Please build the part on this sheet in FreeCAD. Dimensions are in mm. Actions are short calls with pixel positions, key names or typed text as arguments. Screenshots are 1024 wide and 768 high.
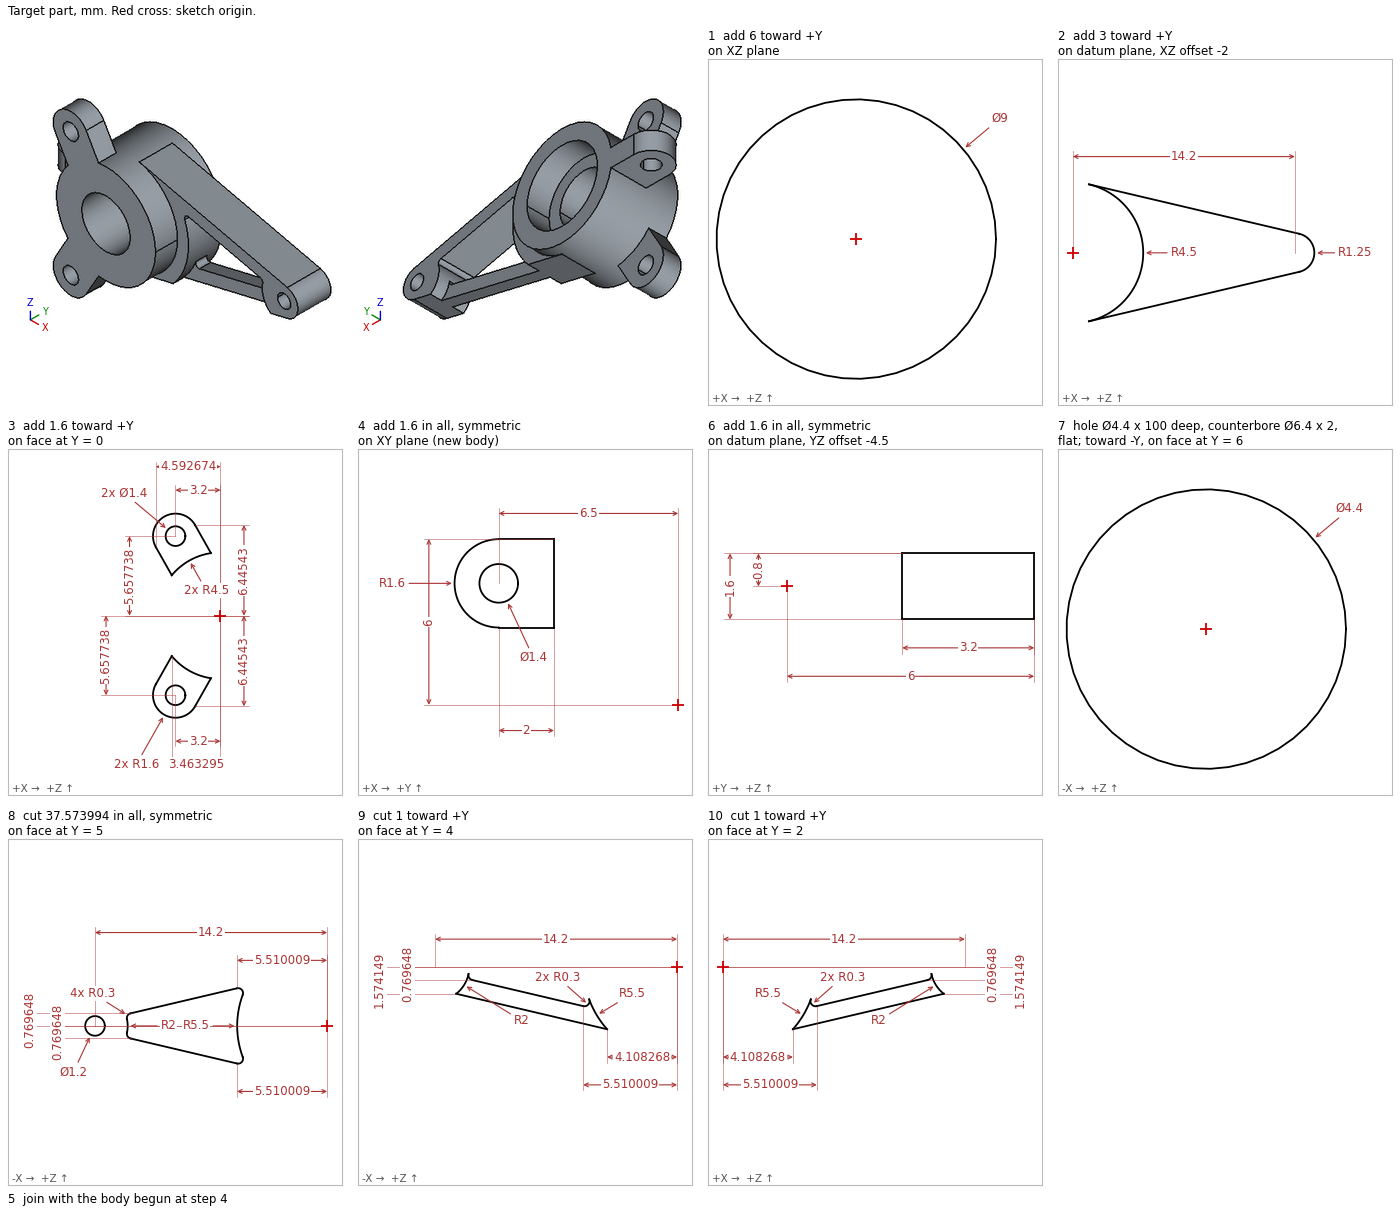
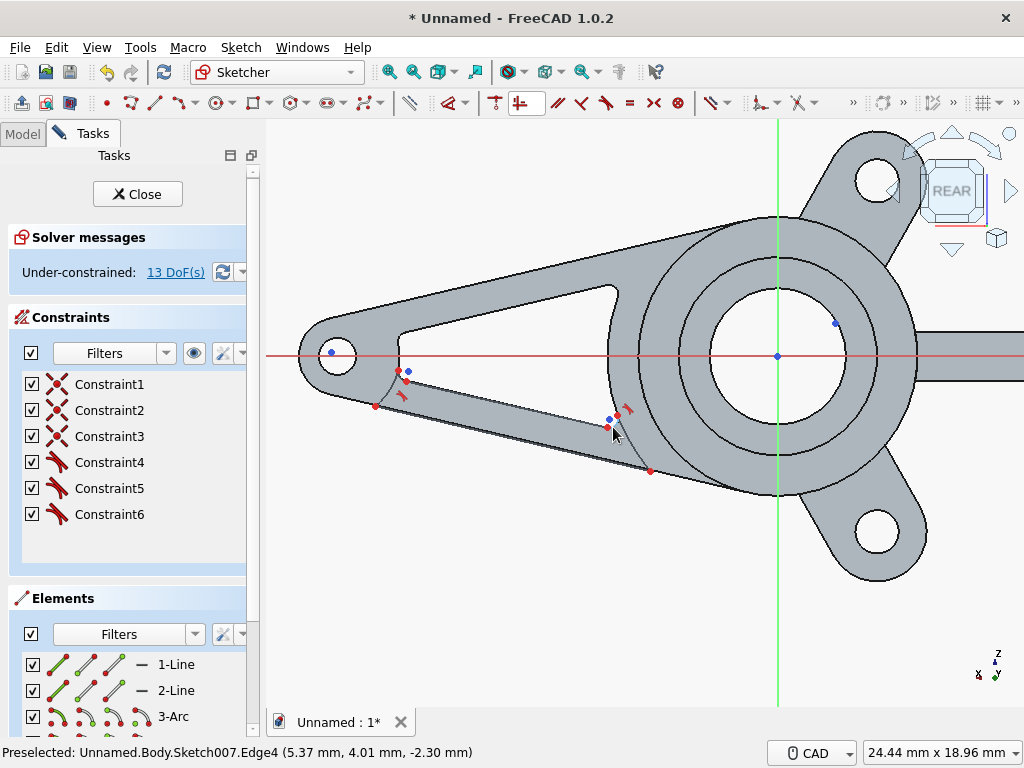
scroll(402, 380, up, 6)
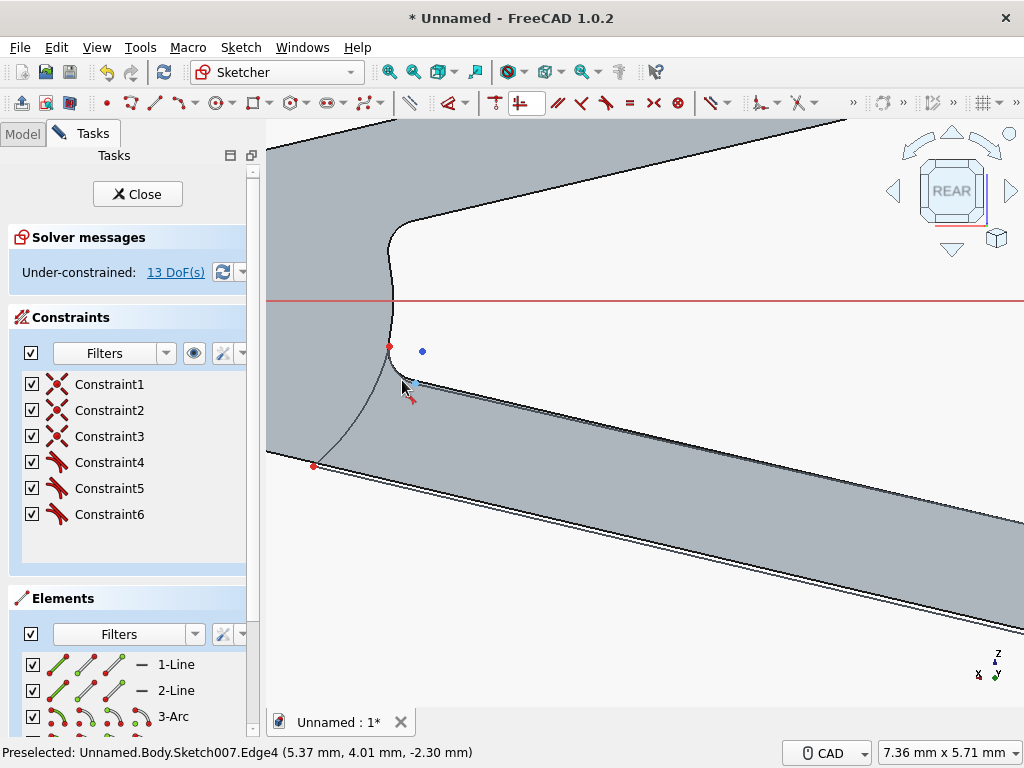
click(402, 377)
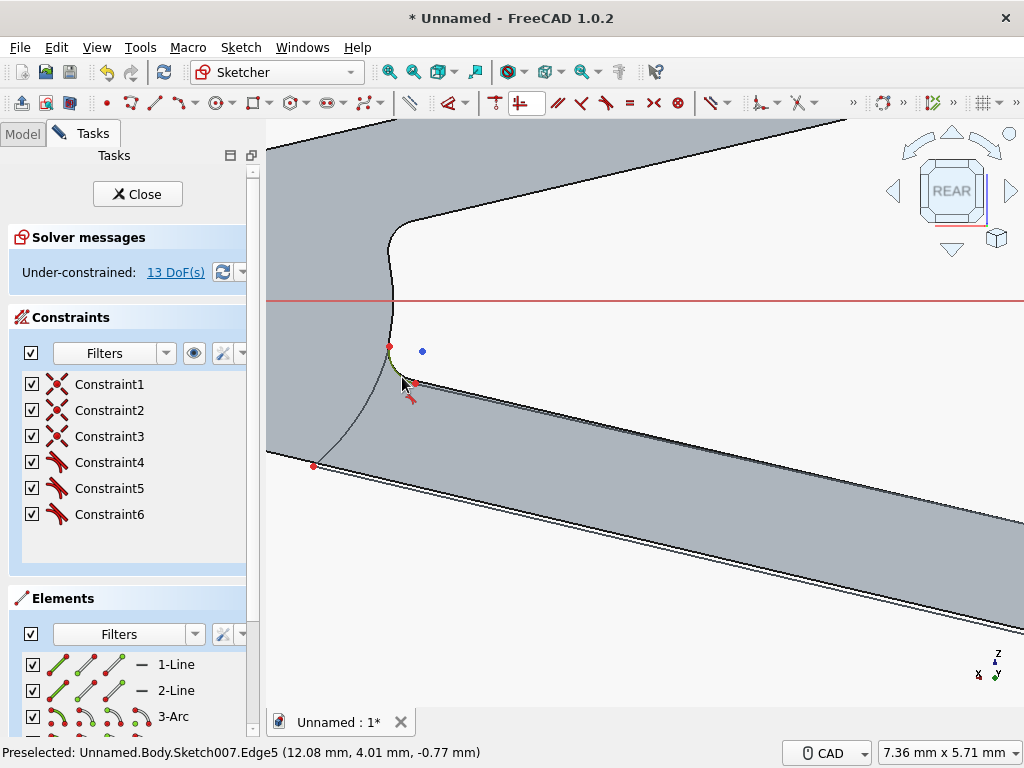
click(344, 436)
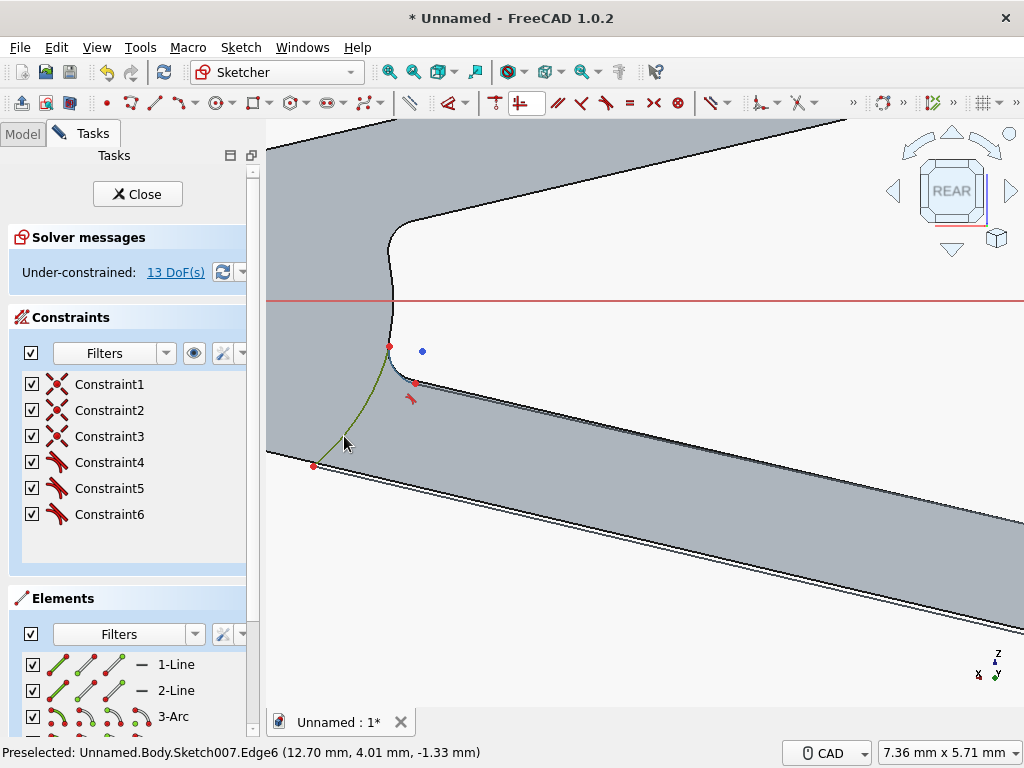
key(t)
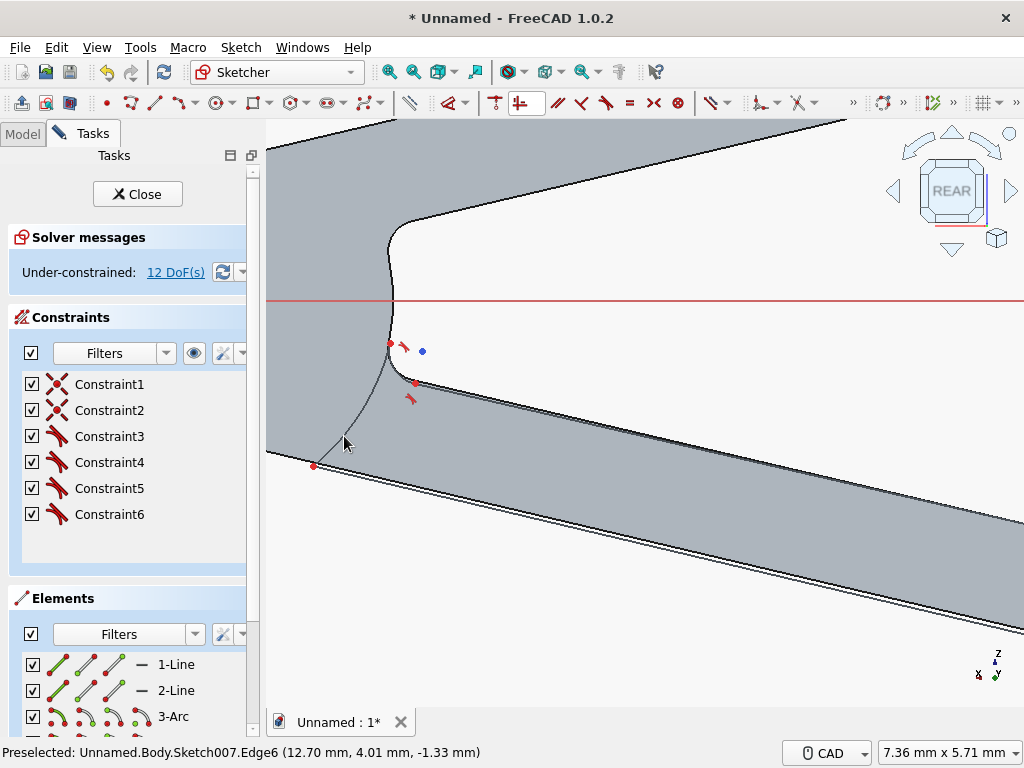
scroll(402, 380, down, 6)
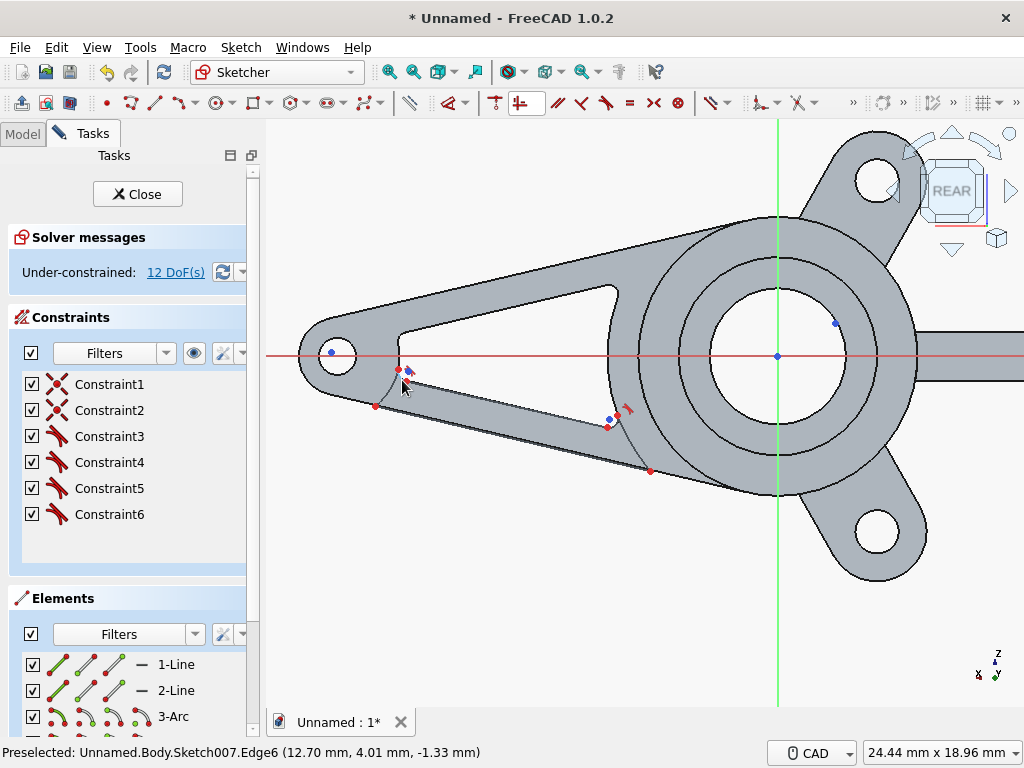
scroll(806, 340, up, 8)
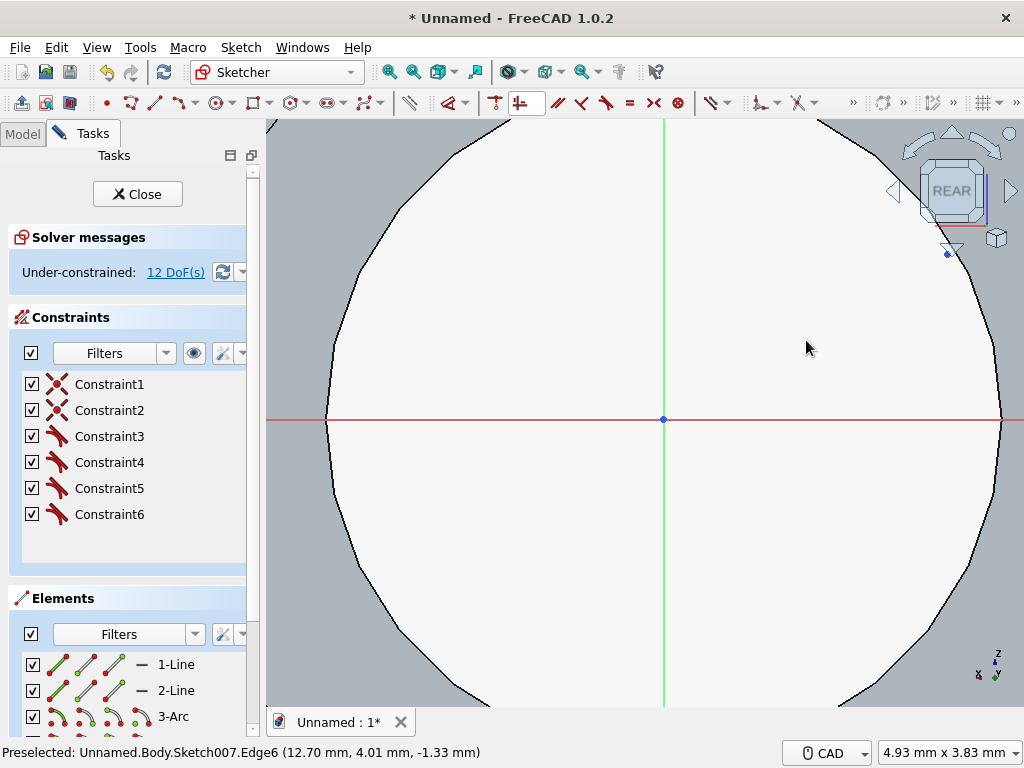
drag(654, 245, 957, 430)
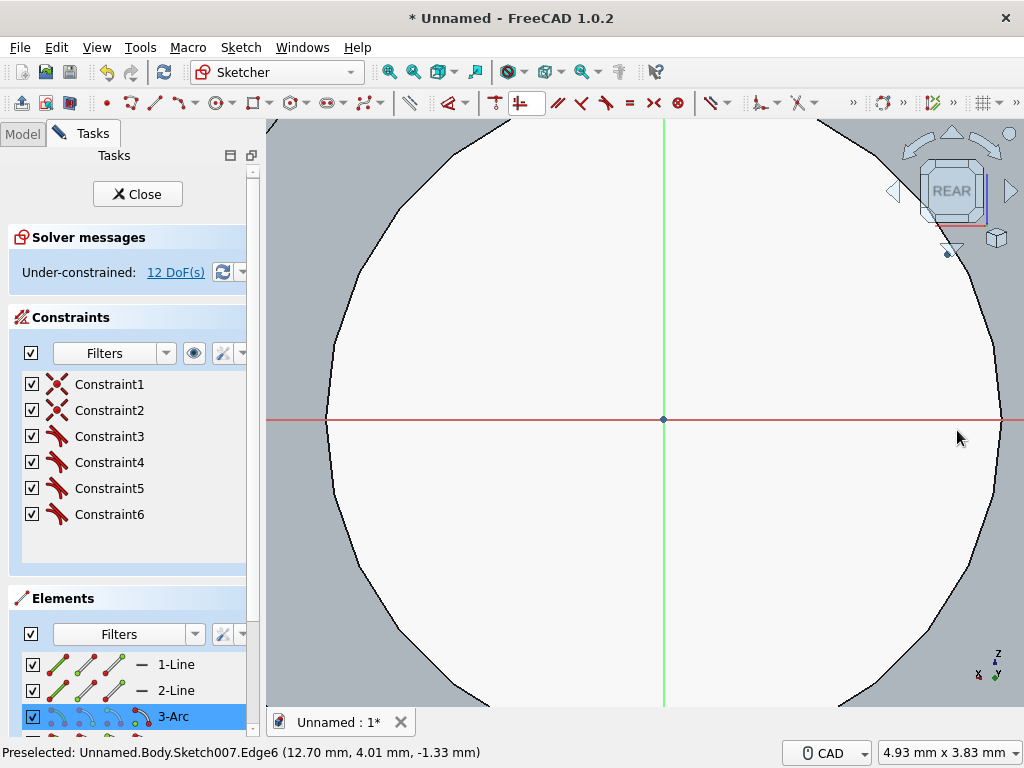
key(c)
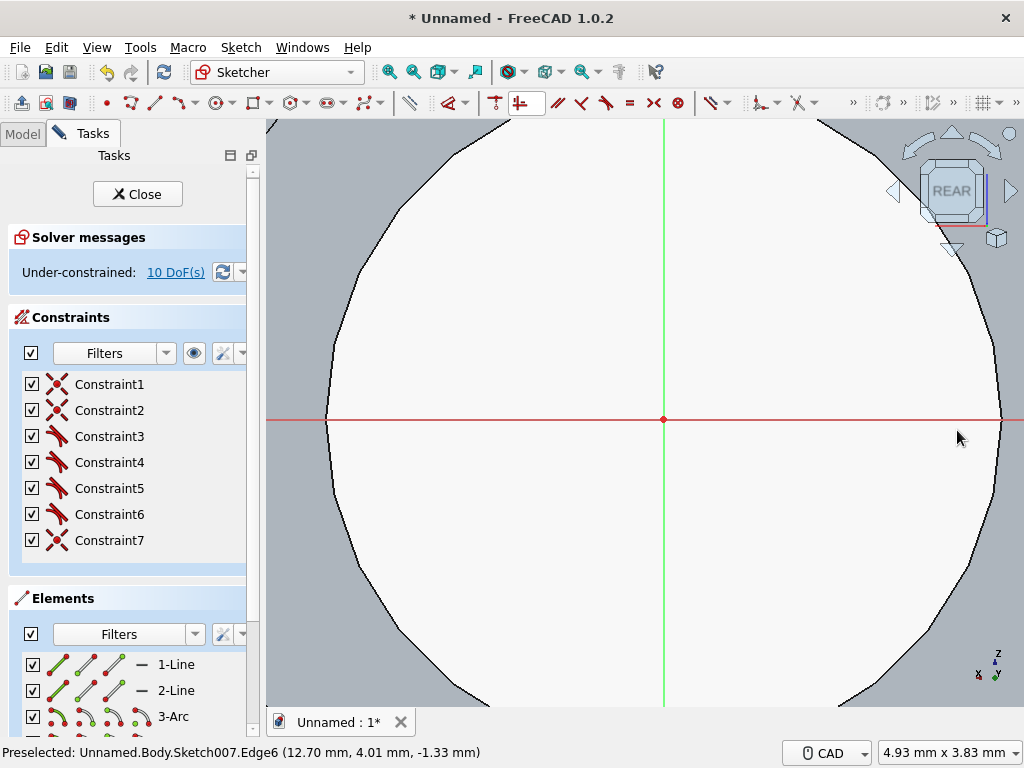
scroll(806, 340, down, 8)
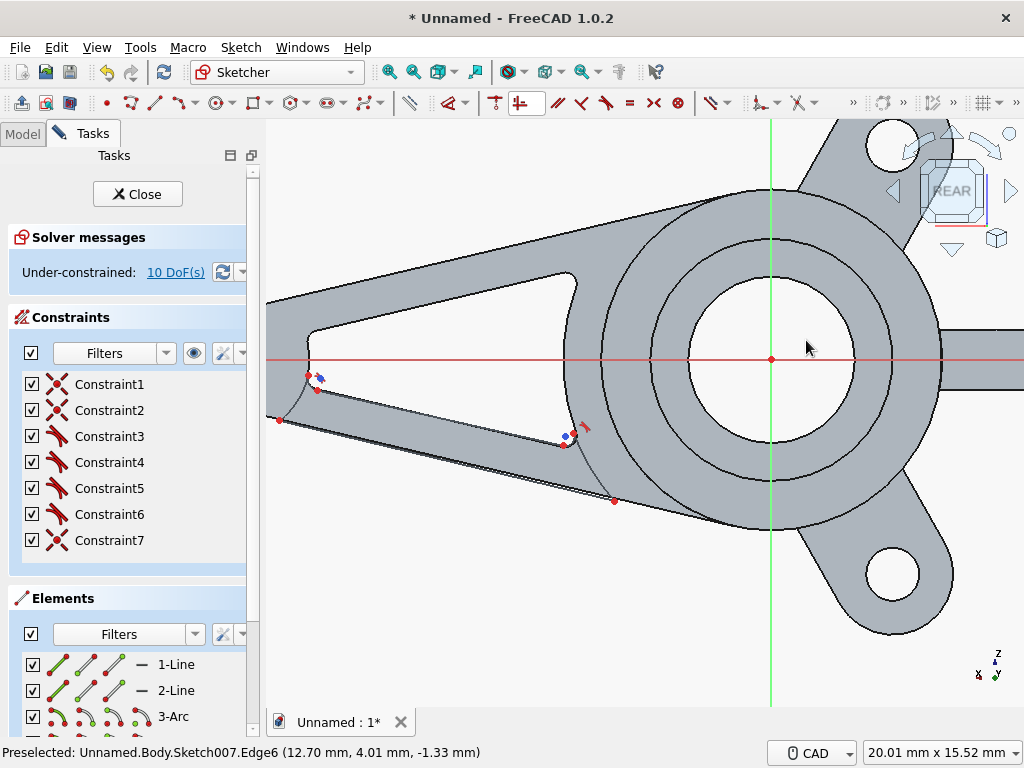
scroll(612, 426, up, 6)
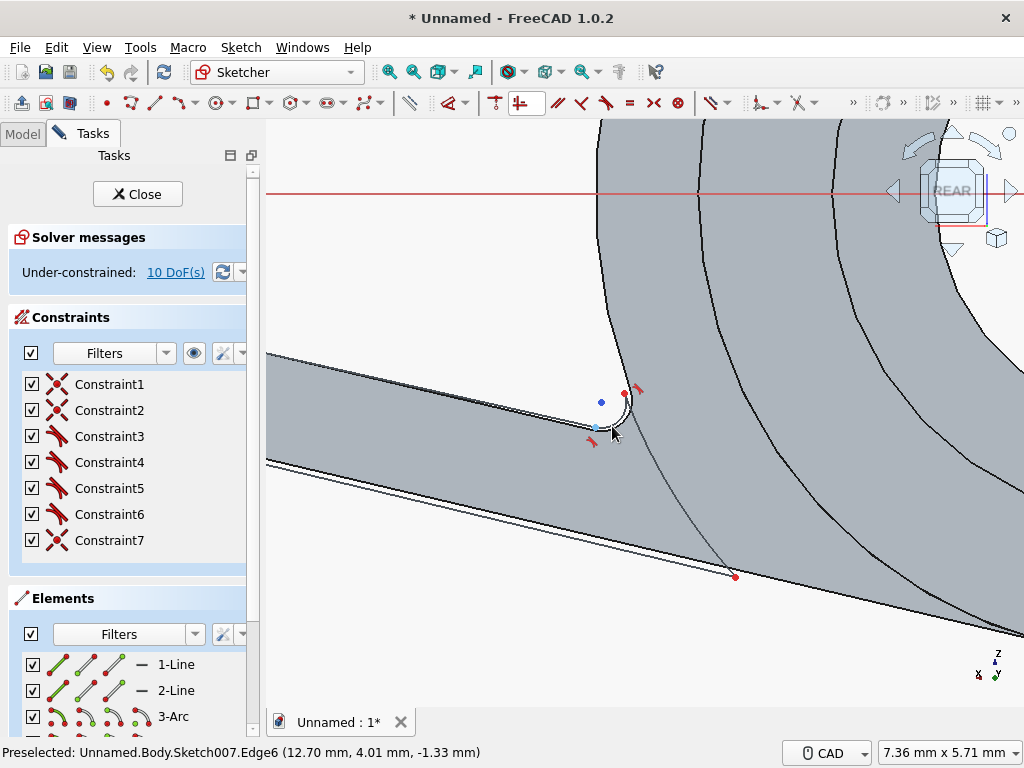
click(612, 426)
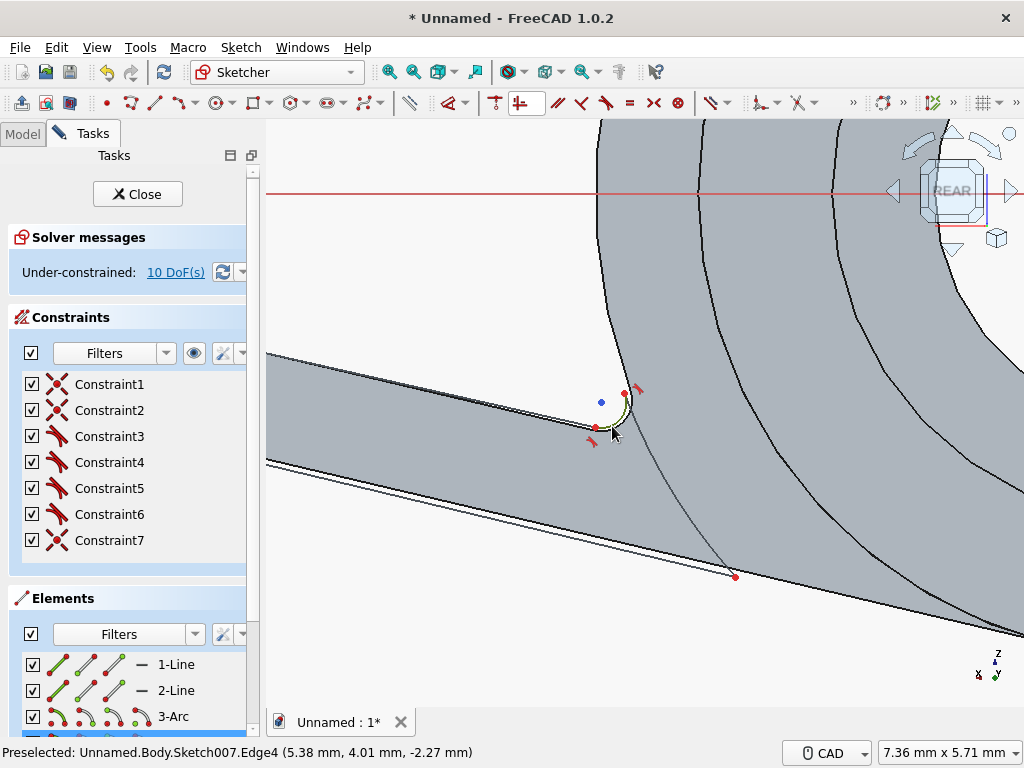
scroll(612, 426, down, 6)